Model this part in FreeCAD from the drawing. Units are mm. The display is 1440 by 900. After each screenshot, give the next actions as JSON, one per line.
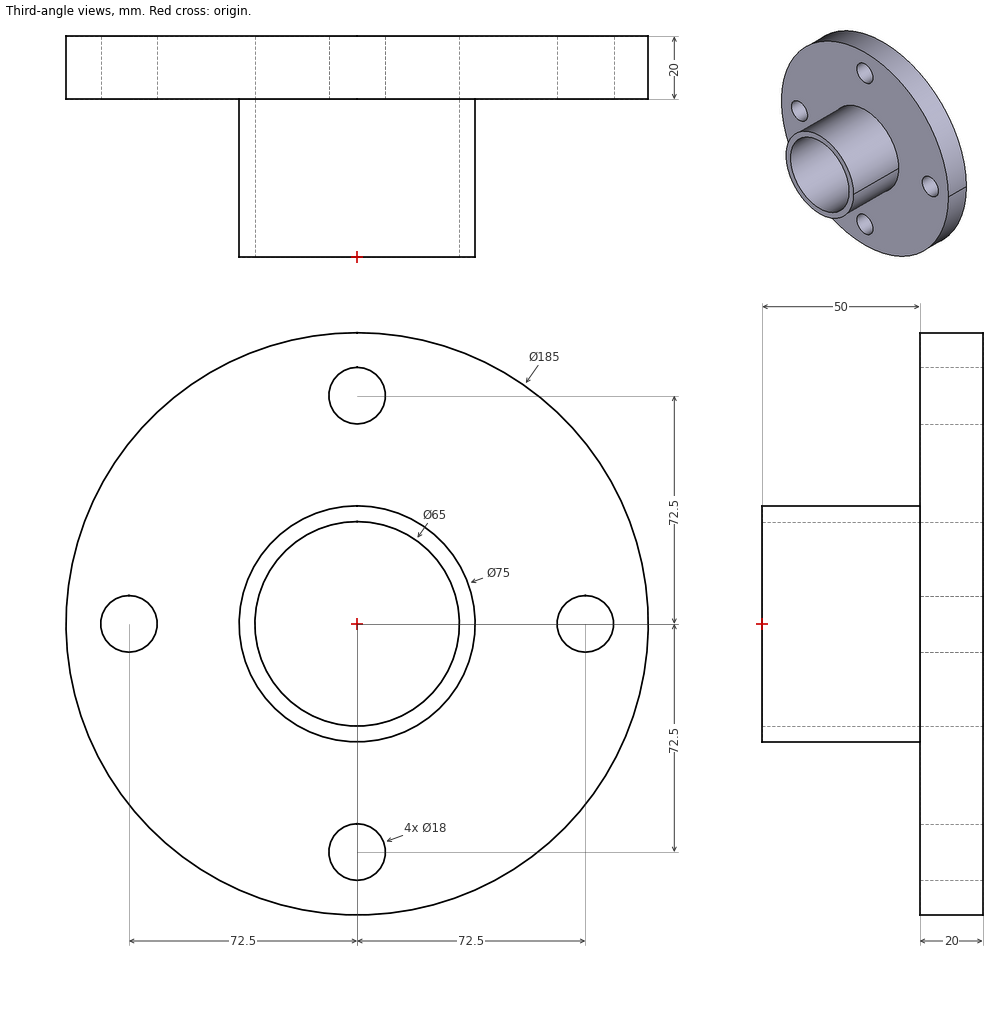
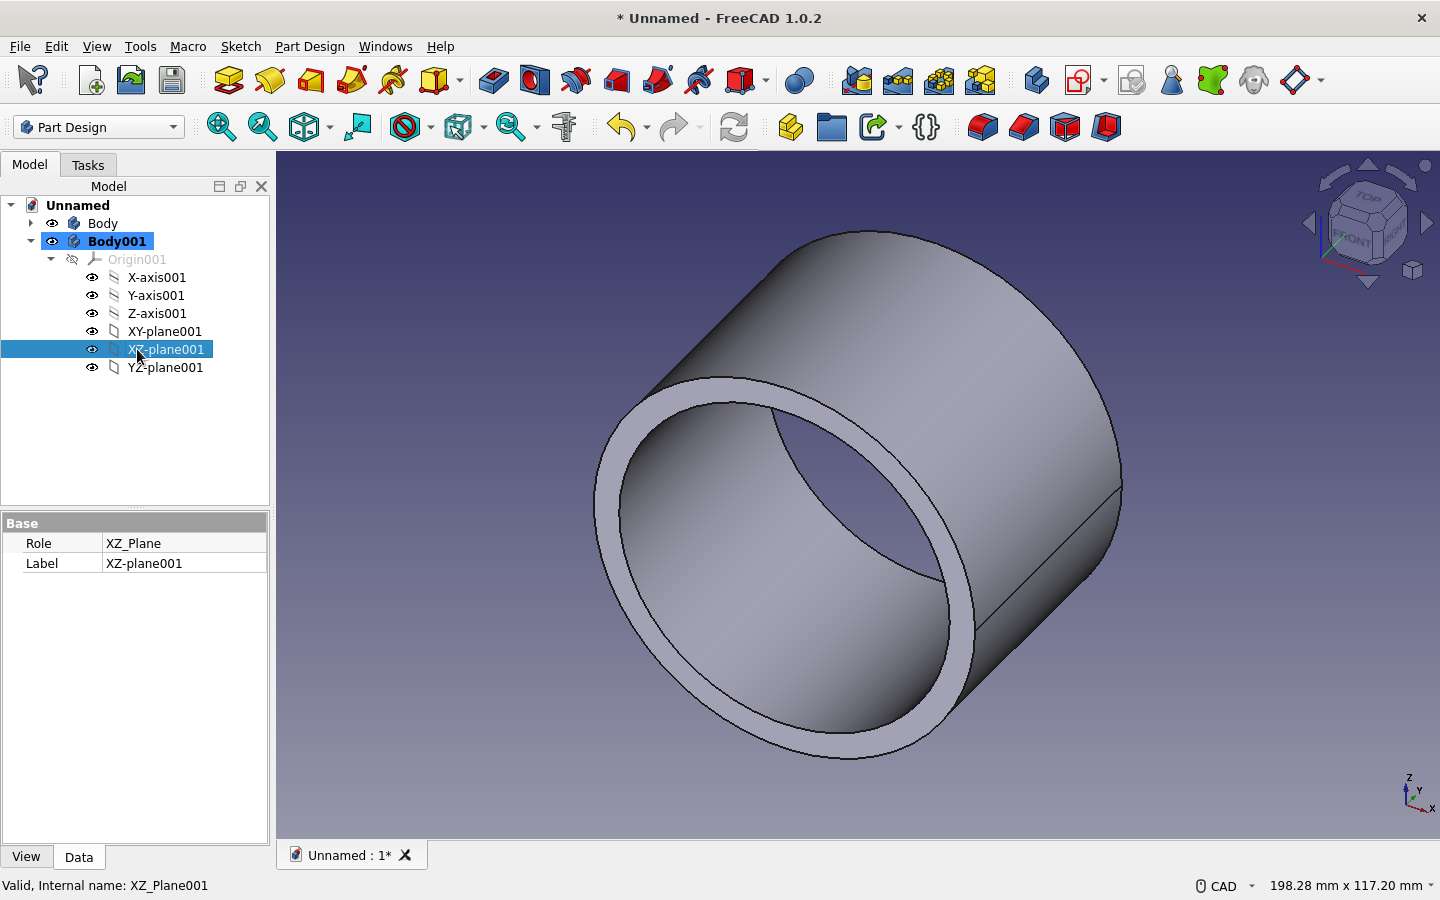
{"action": "left_click", "coordinate": [1294, 80]}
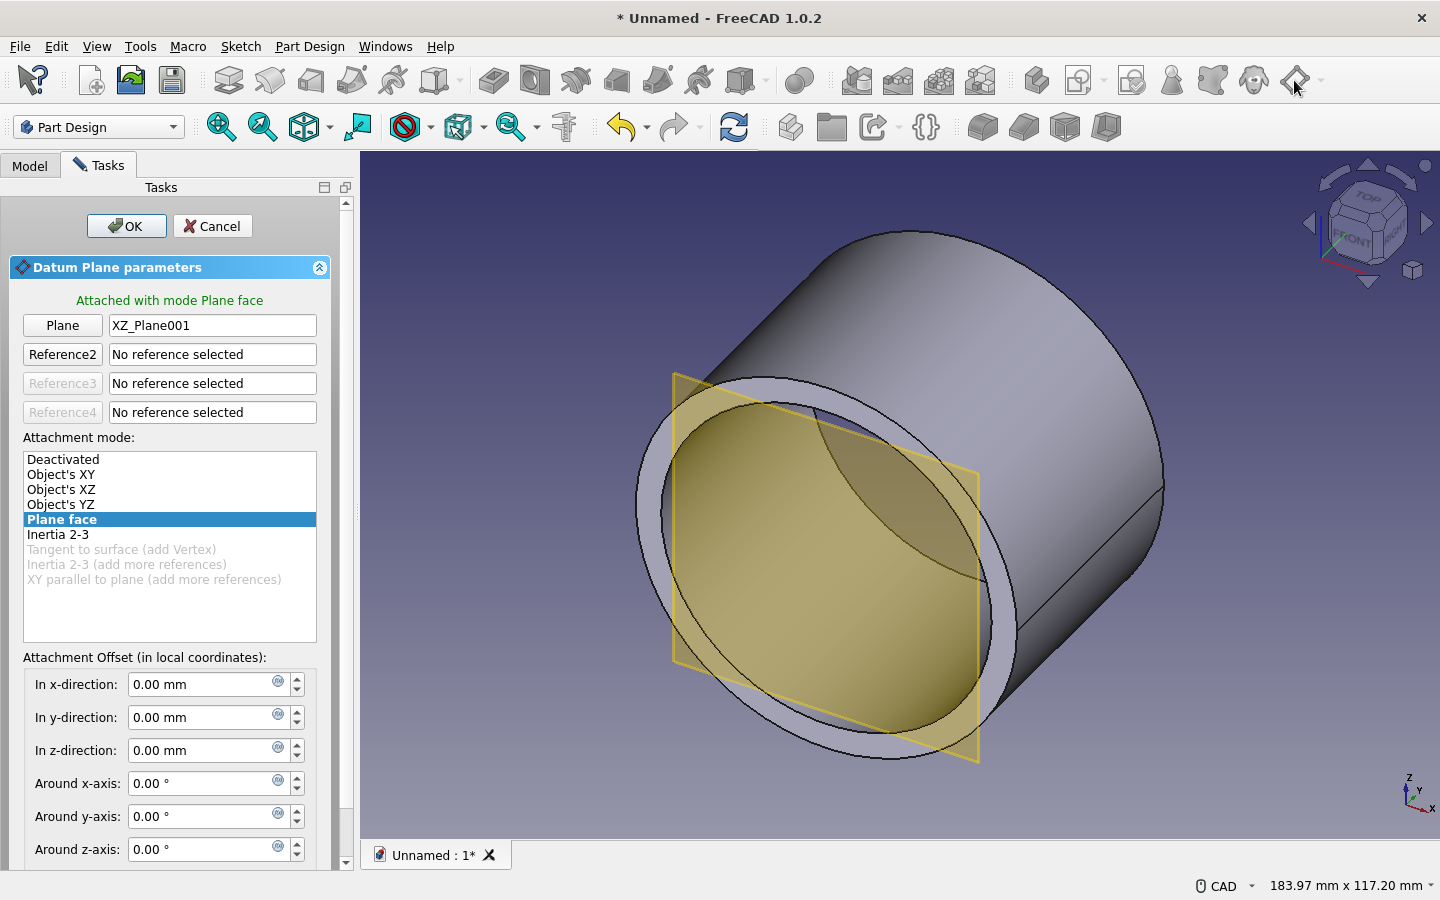
{"action": "triple_click", "coordinate": [210, 750]}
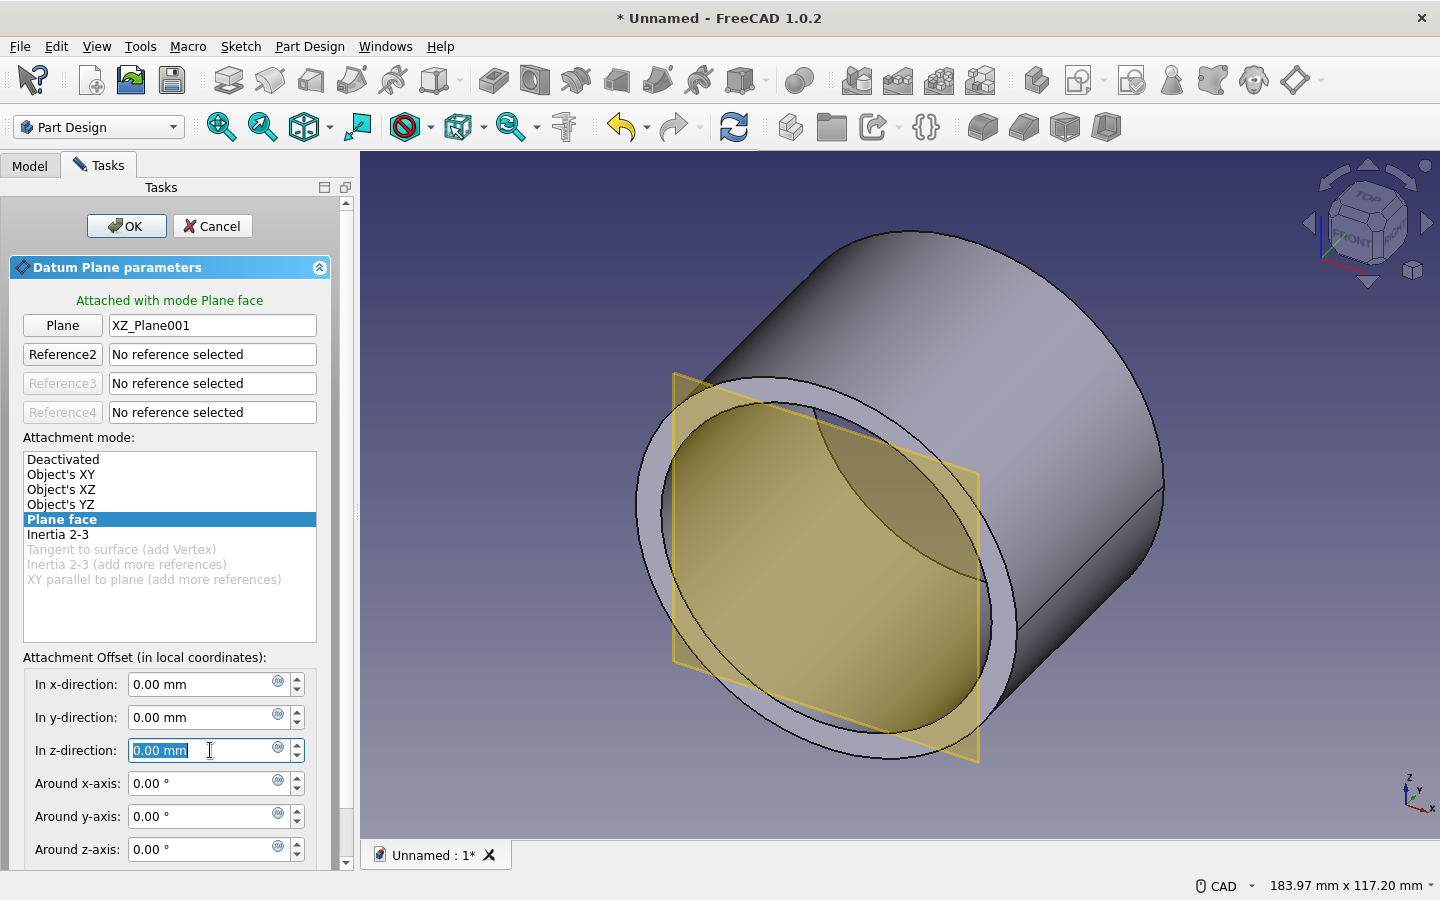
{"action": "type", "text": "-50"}
{"action": "key", "text": "Tab"}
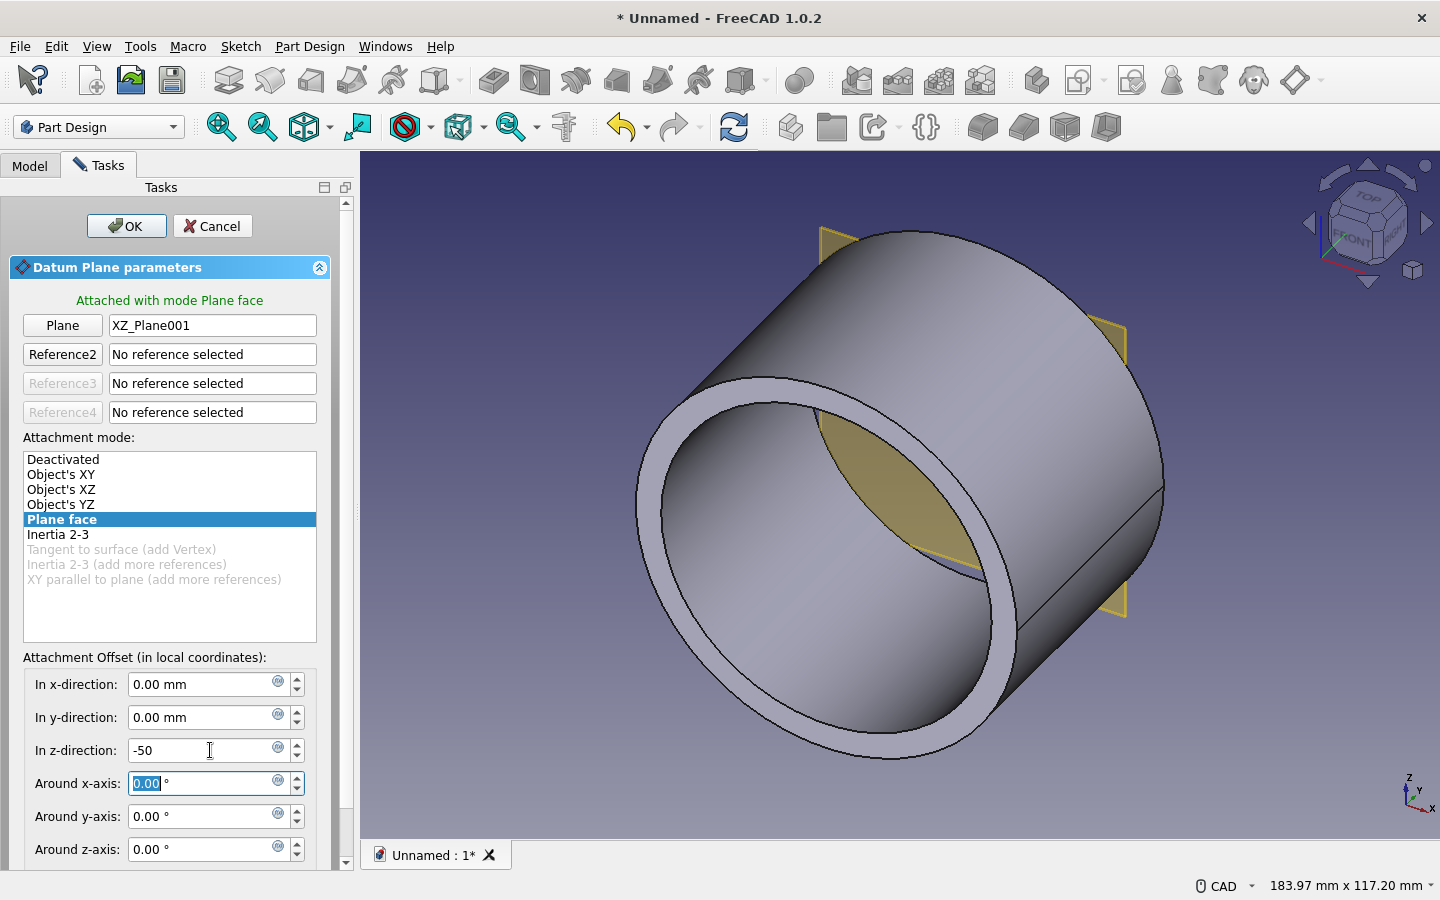
{"action": "left_click", "coordinate": [127, 226]}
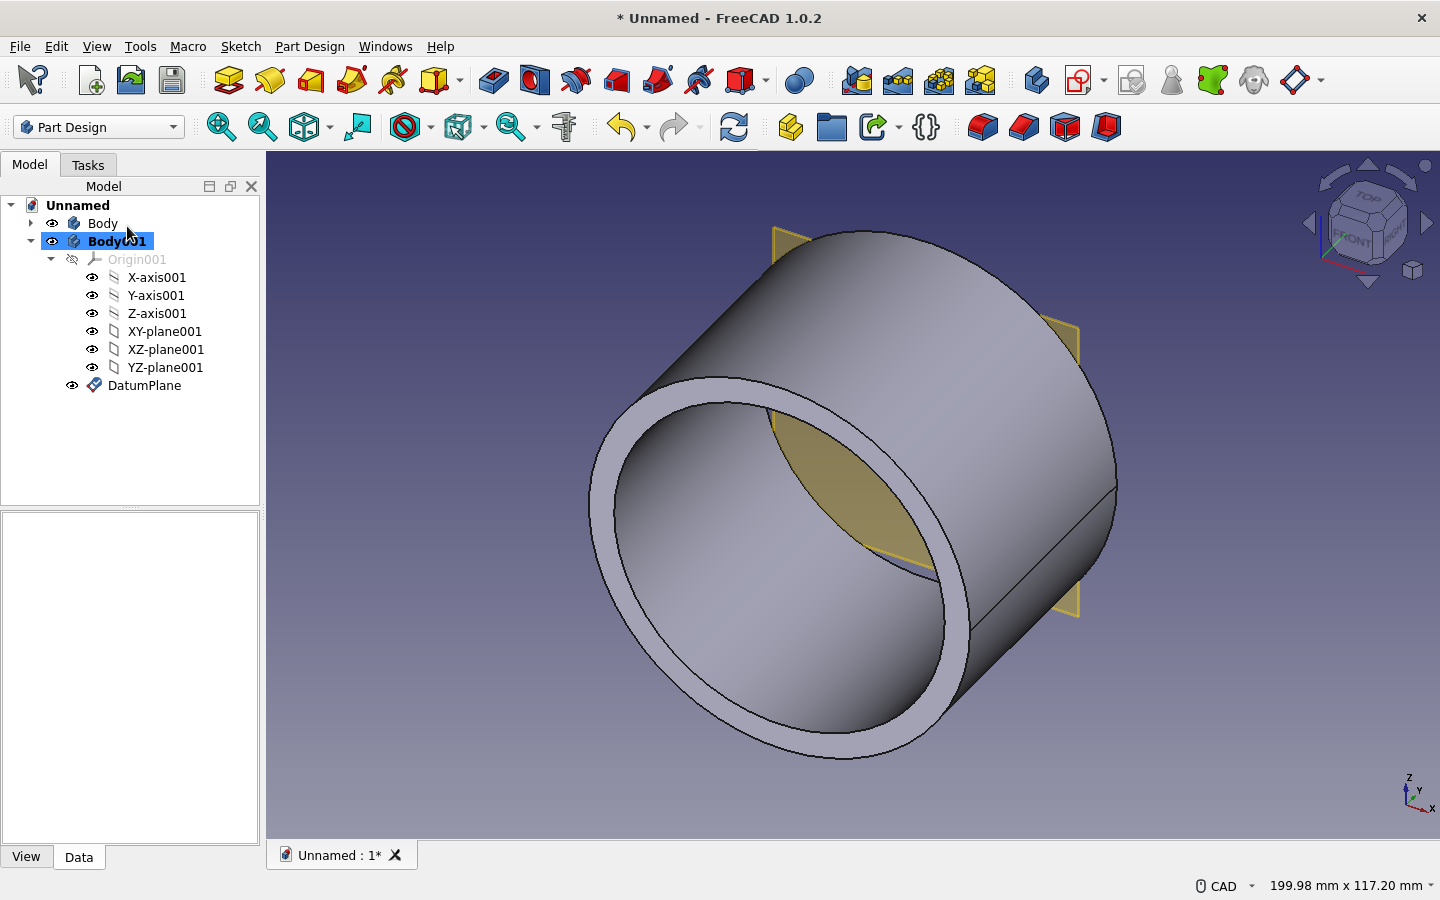
{"action": "left_click", "coordinate": [117, 385]}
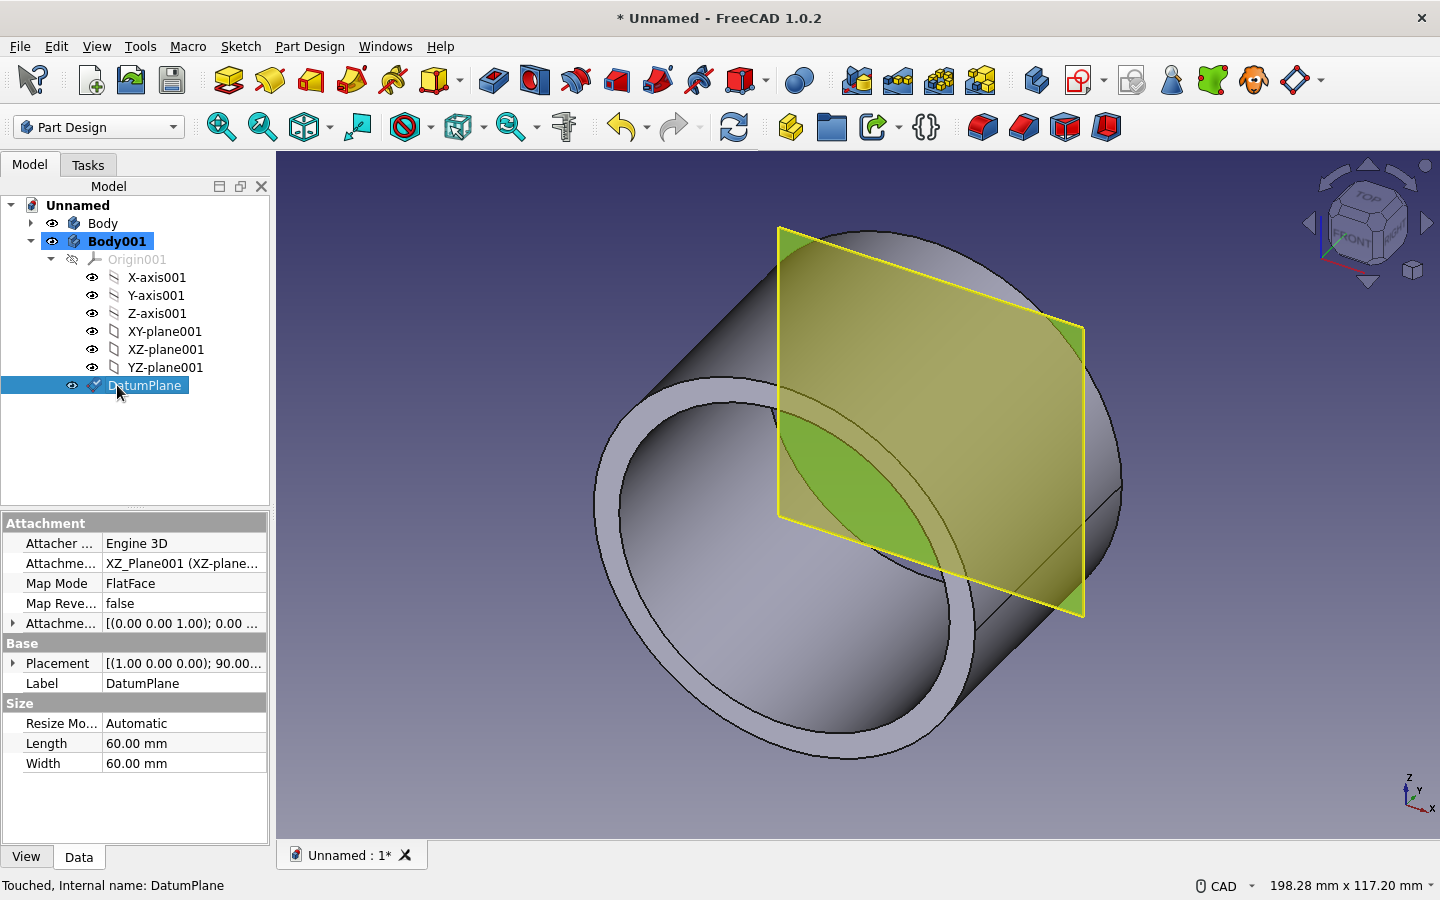
{"action": "left_click", "coordinate": [1078, 80]}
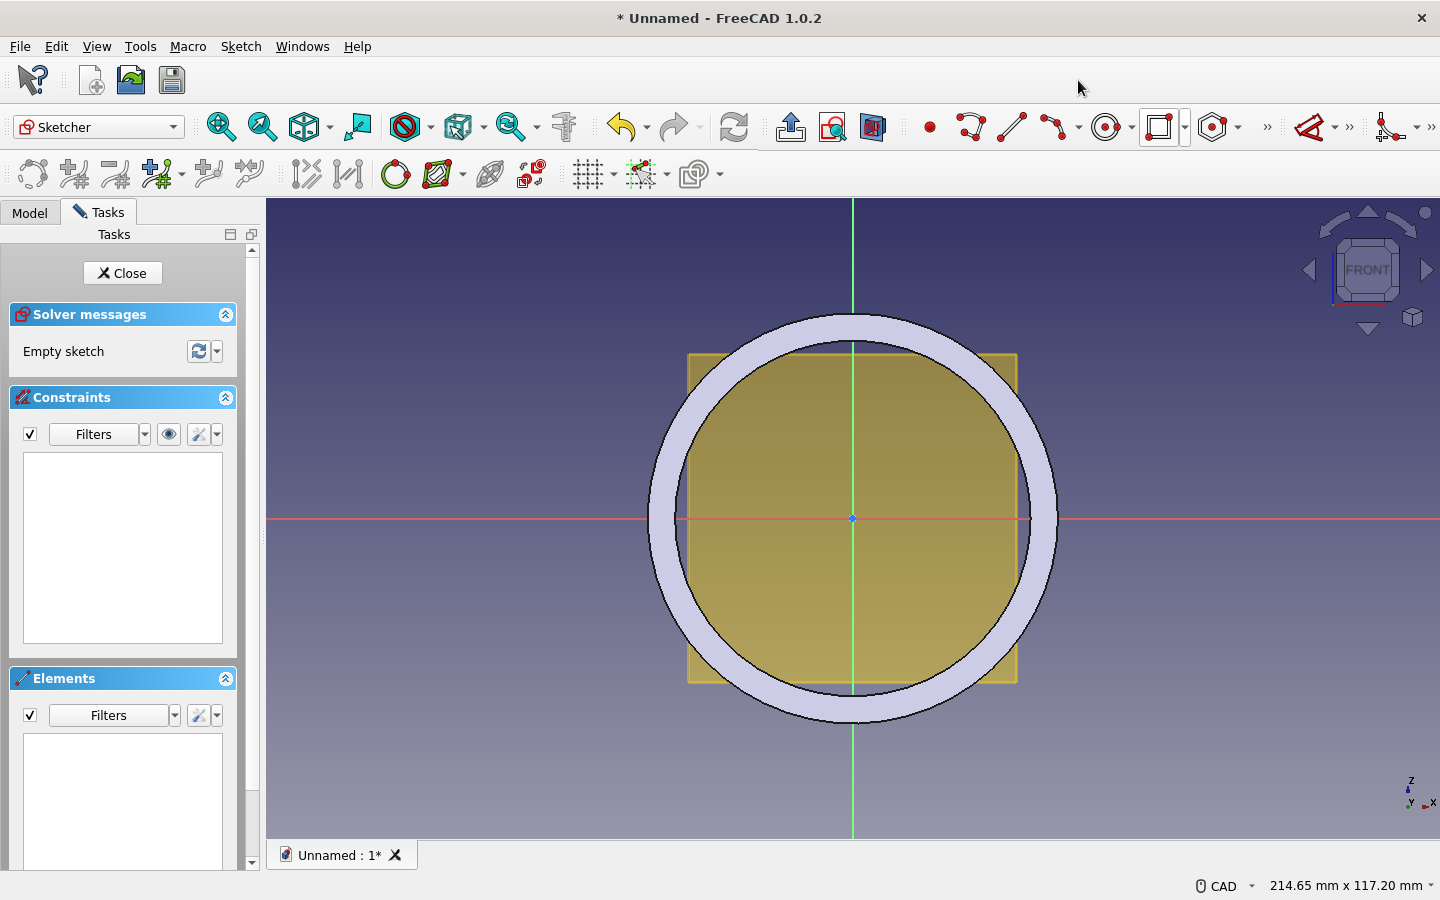
{"action": "scroll", "coordinate": [729, 518], "scroll_direction": "down", "scroll_amount": 4}